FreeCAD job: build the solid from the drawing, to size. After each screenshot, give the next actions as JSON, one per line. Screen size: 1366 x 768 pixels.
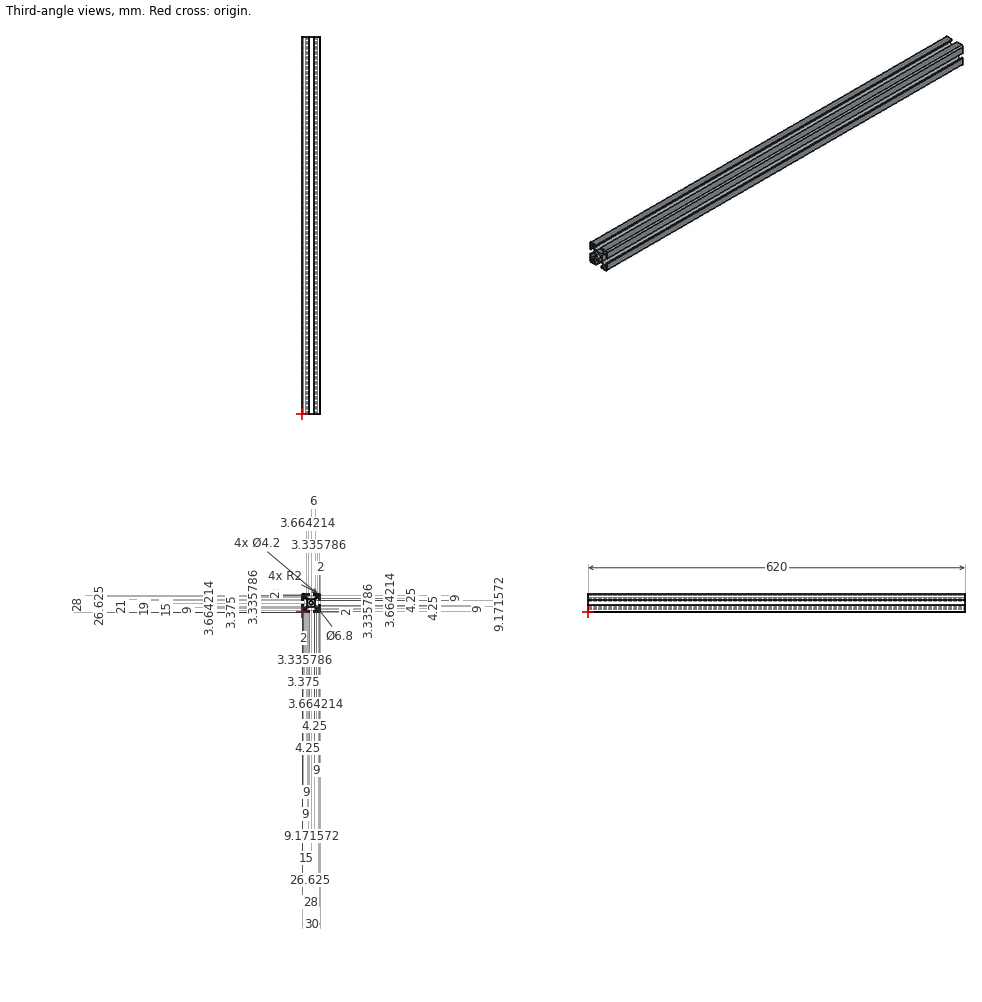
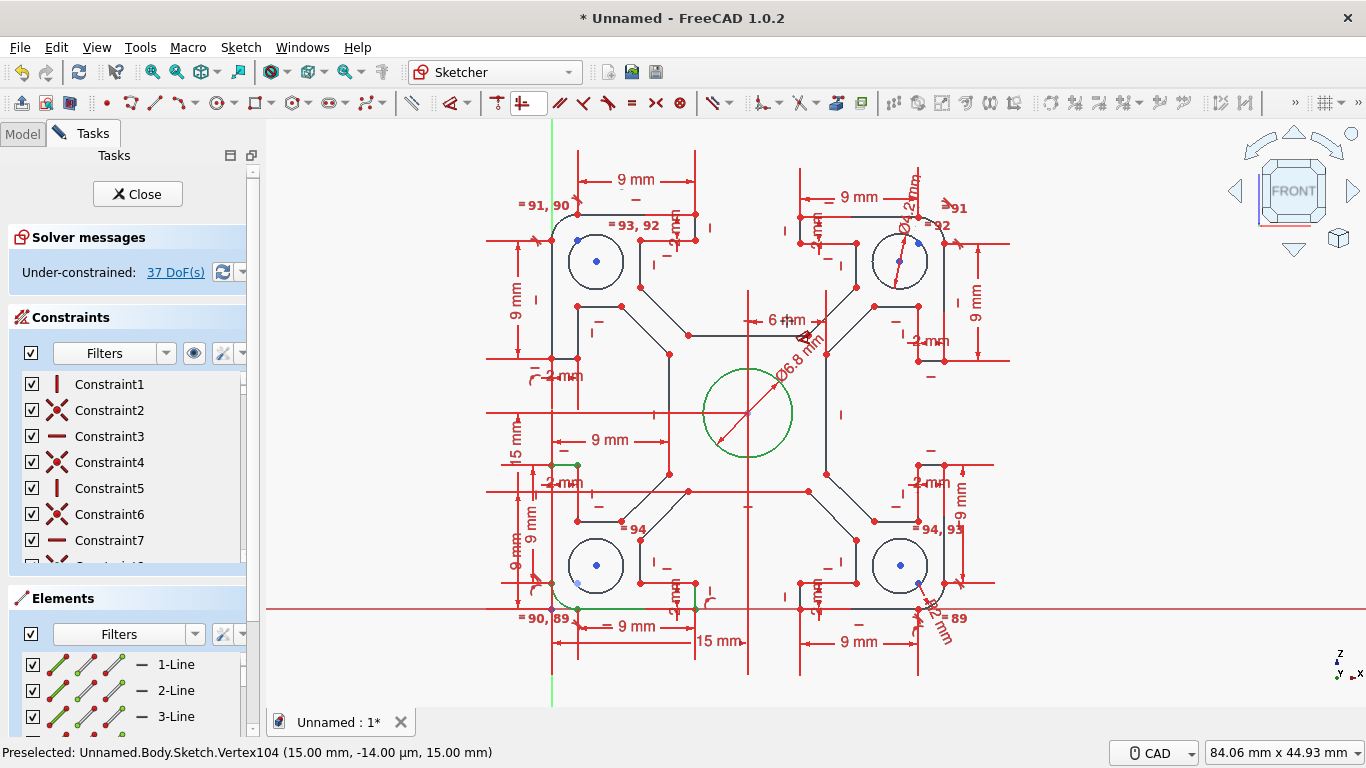
{"action": "left_click", "coordinate": [944, 244]}
{"action": "left_click", "coordinate": [748, 210]}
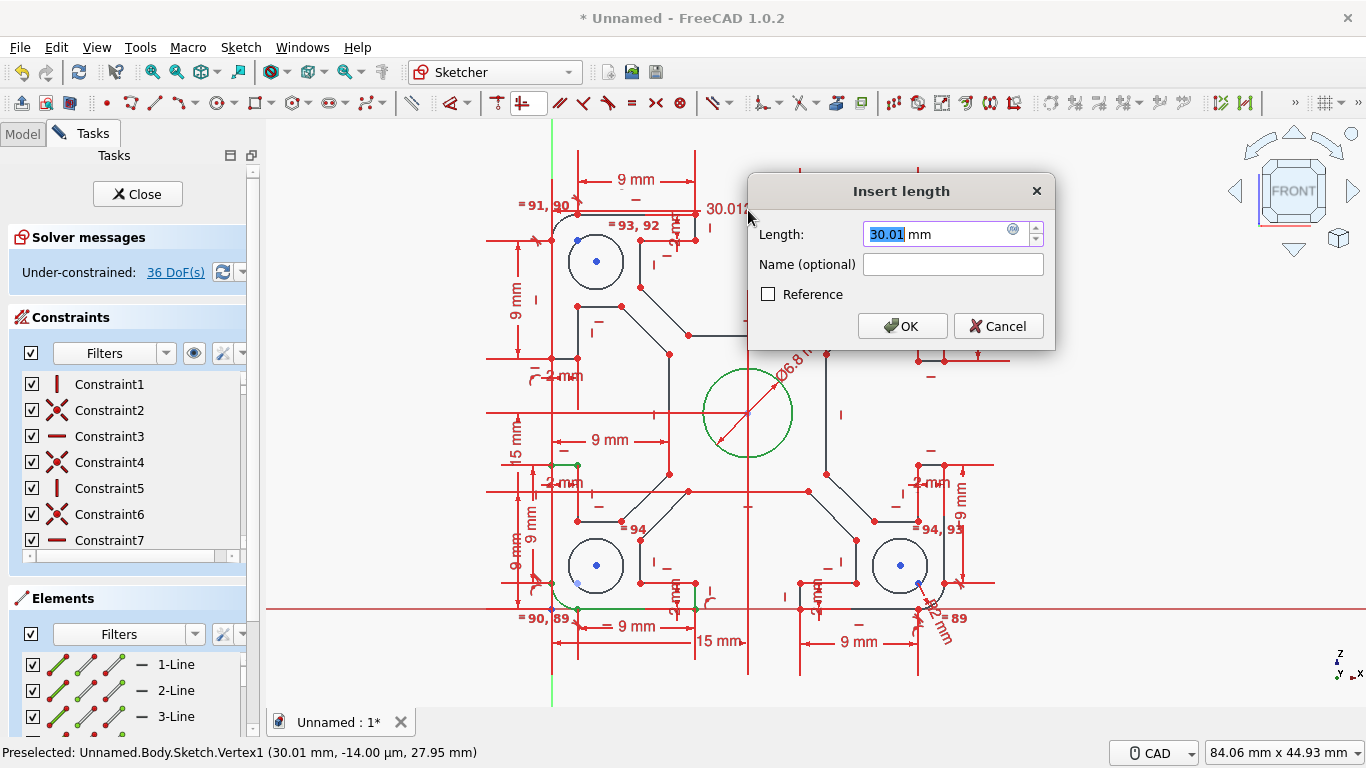
{"action": "type", "text": "30"}
{"action": "key", "text": "Return"}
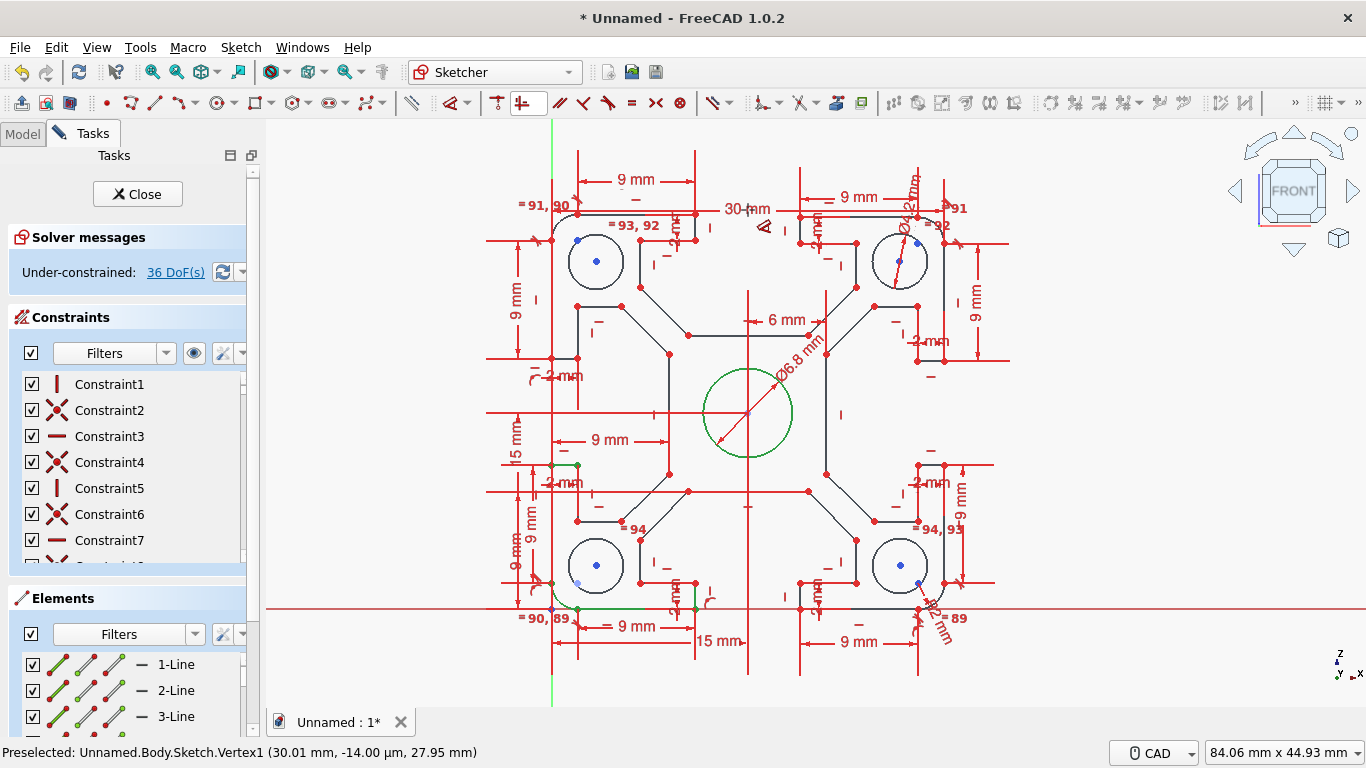
{"action": "left_click", "coordinate": [944, 244]}
{"action": "left_click", "coordinate": [518, 342]}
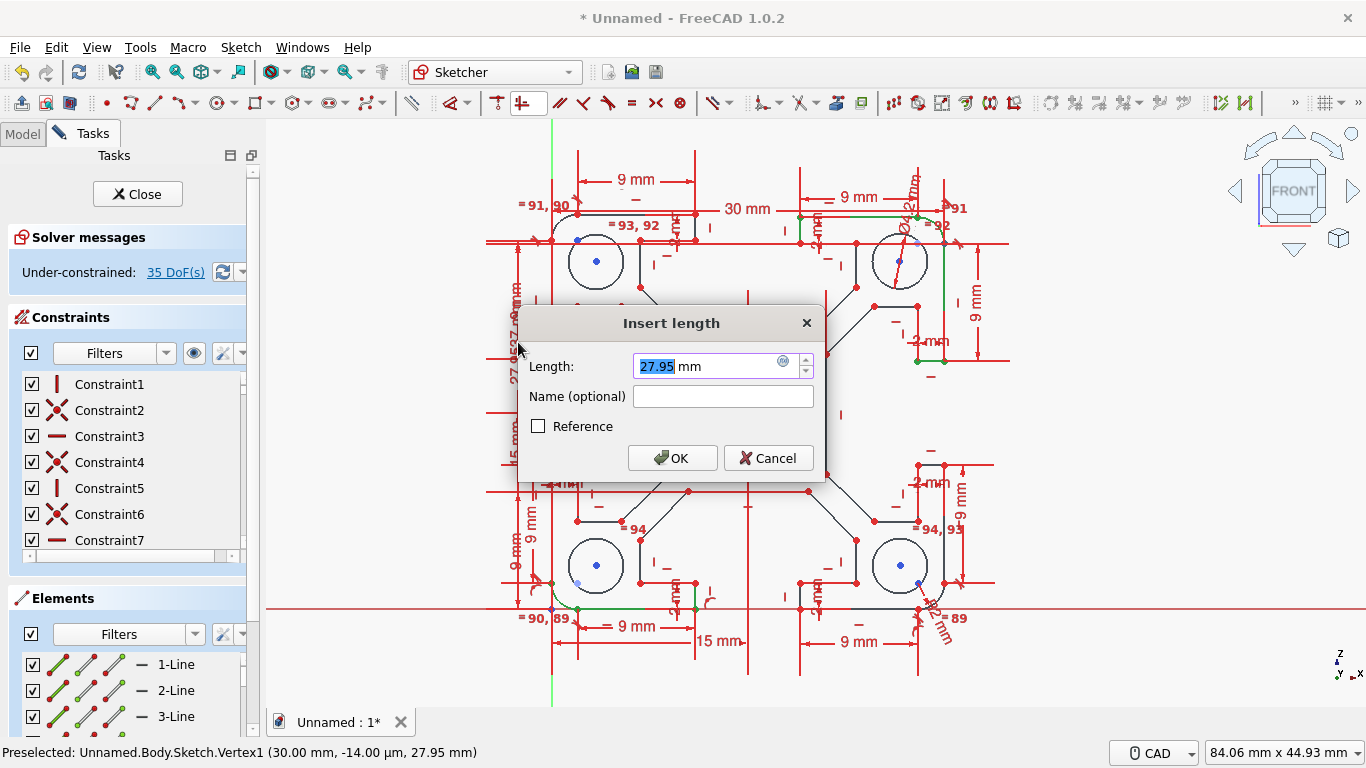
{"action": "type", "text": "28"}
{"action": "key", "text": "Return"}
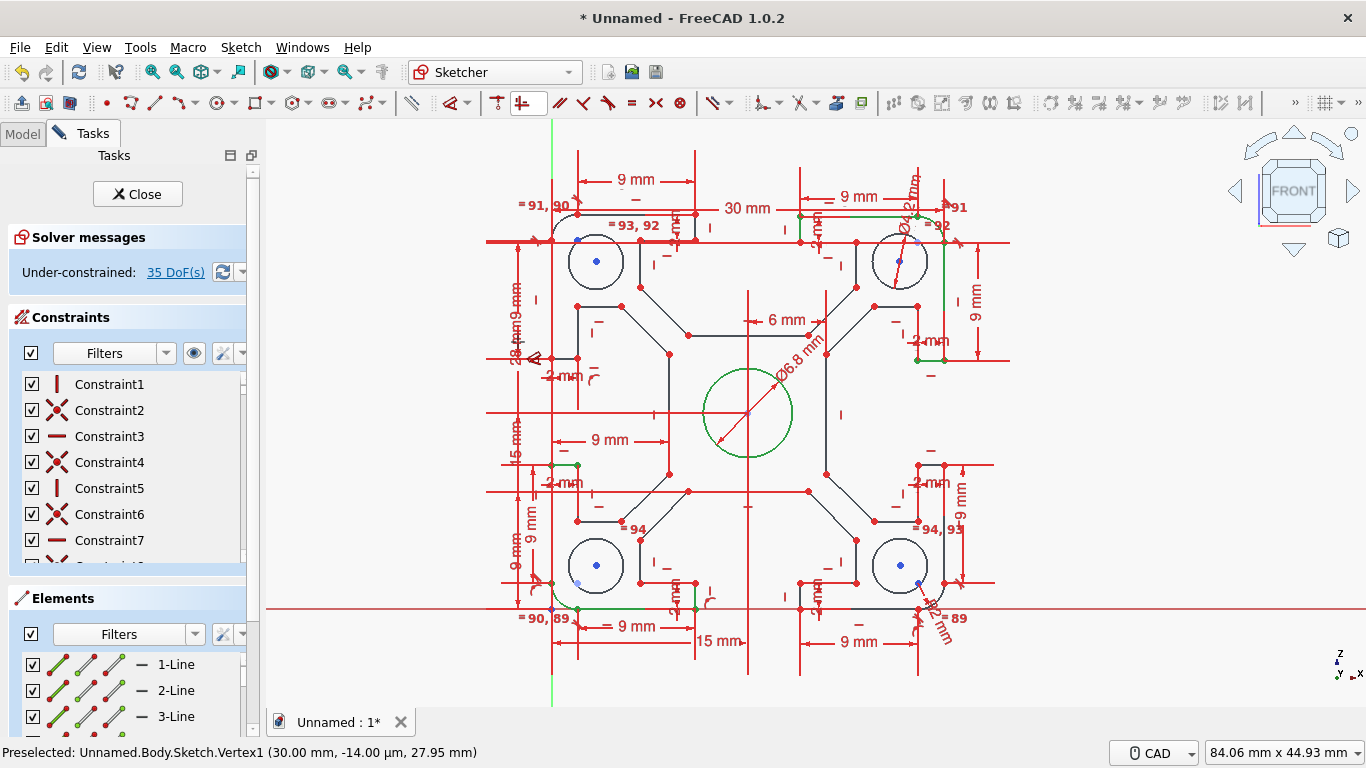
{"action": "left_click", "coordinate": [918, 522]}
{"action": "left_click", "coordinate": [735, 667]}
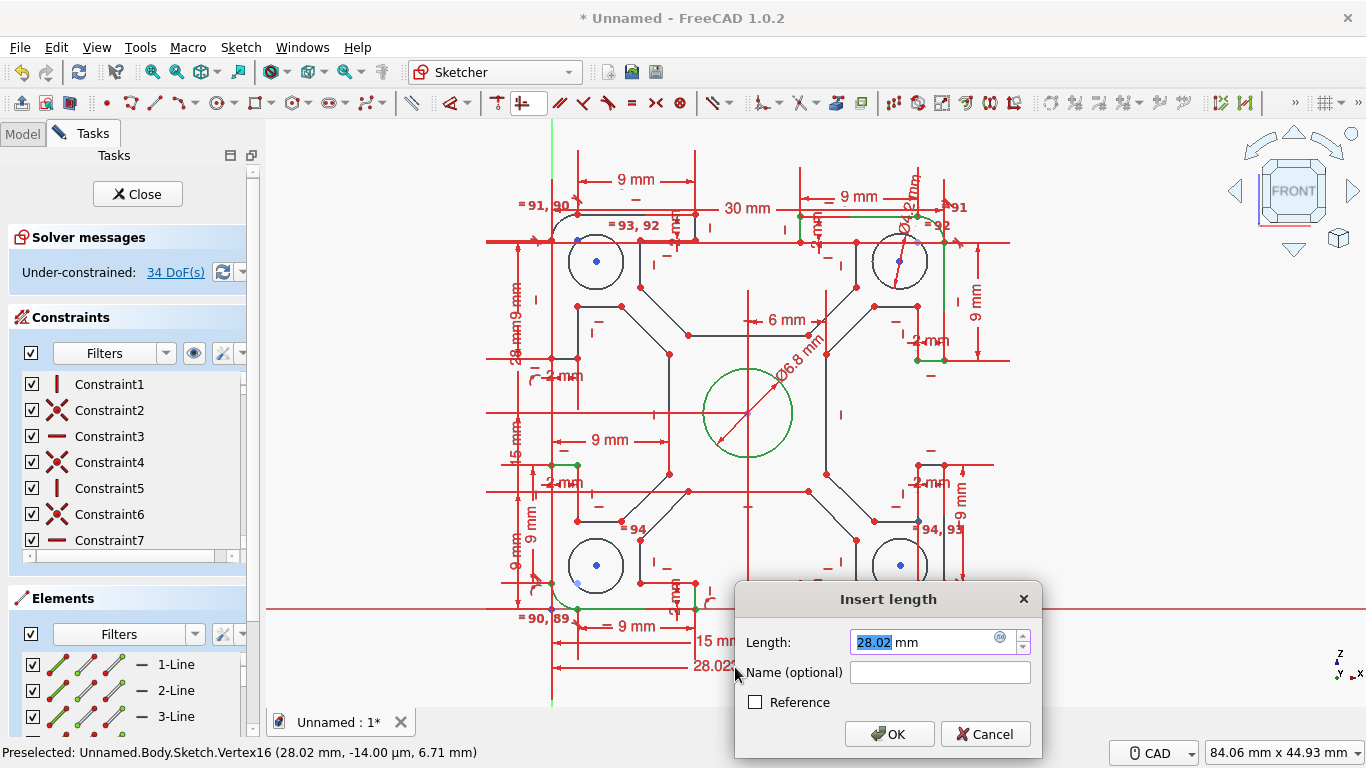
{"action": "type", "text": "28"}
{"action": "key", "text": "Return"}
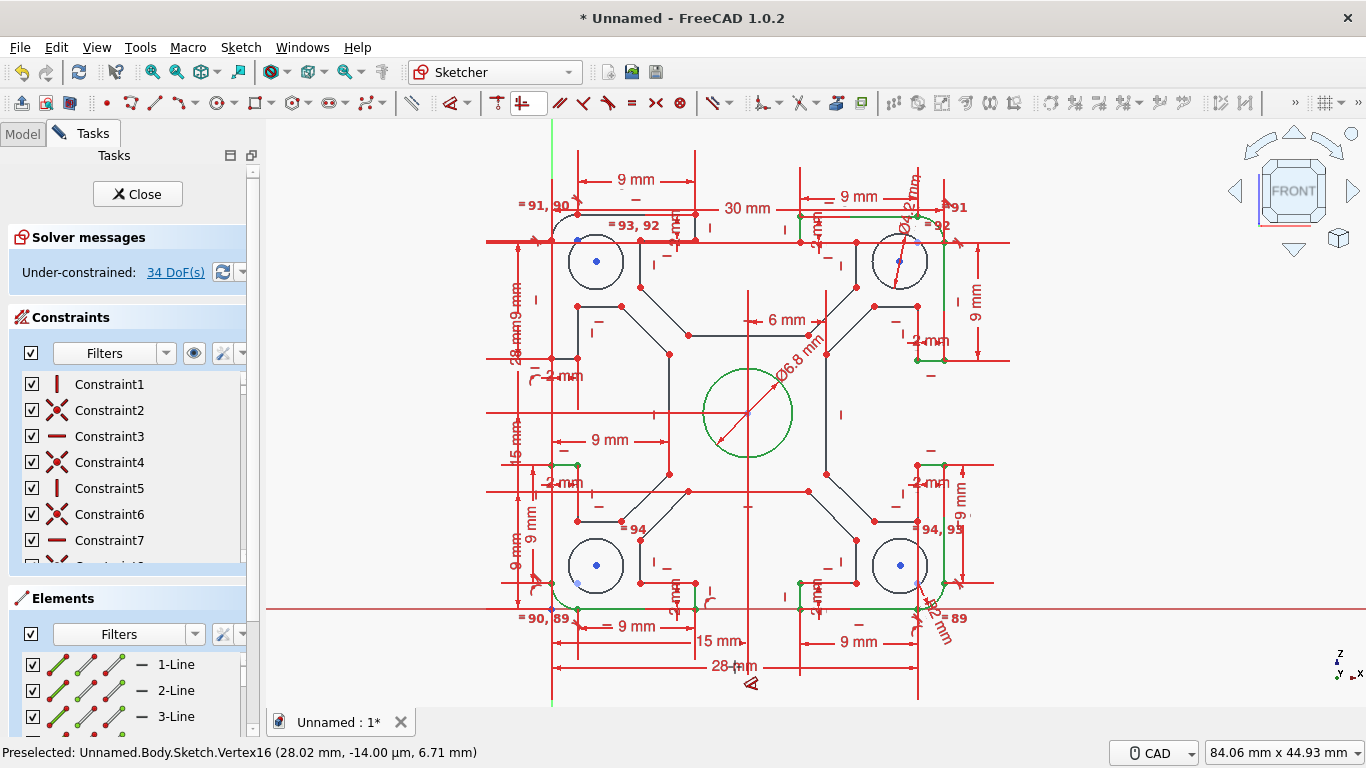
{"action": "left_click", "coordinate": [578, 359]}
{"action": "left_click", "coordinate": [518, 572]}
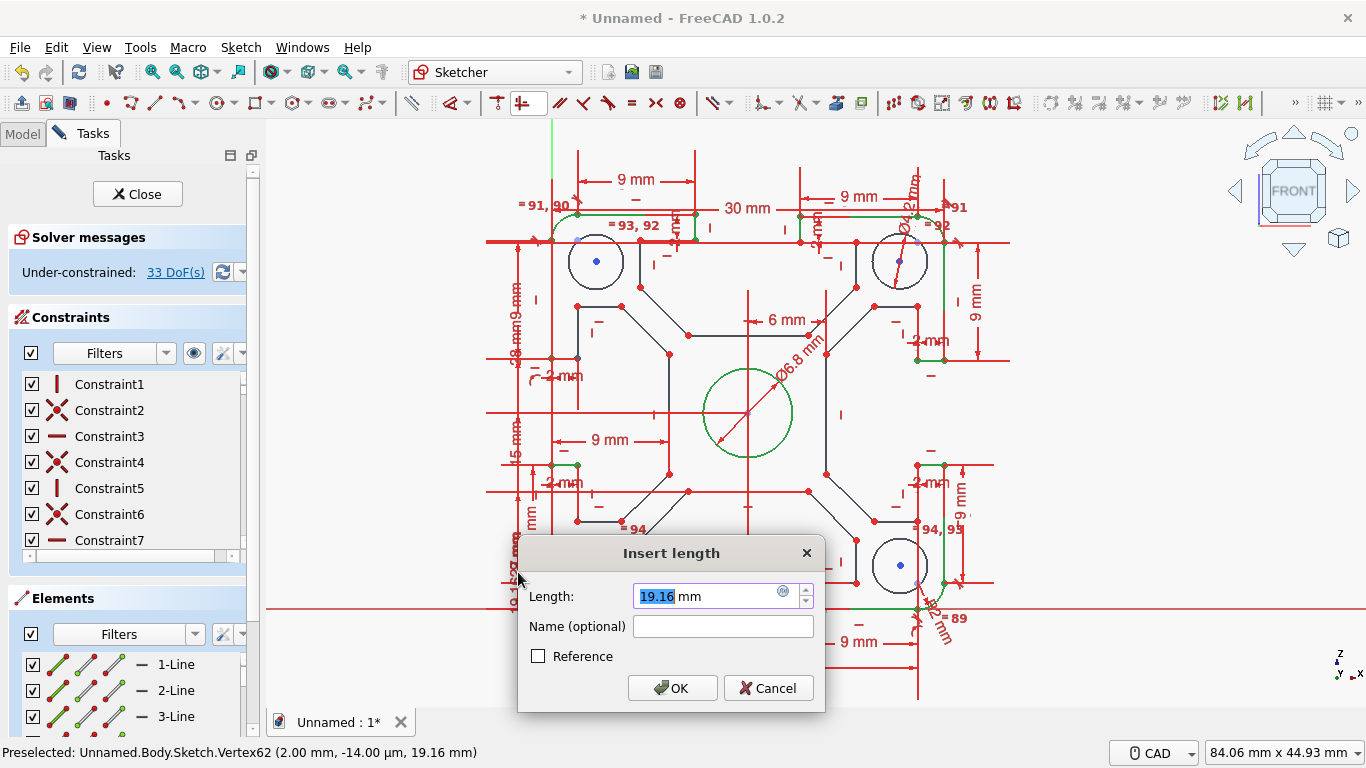
{"action": "type", "text": "19"}
{"action": "key", "text": "Return"}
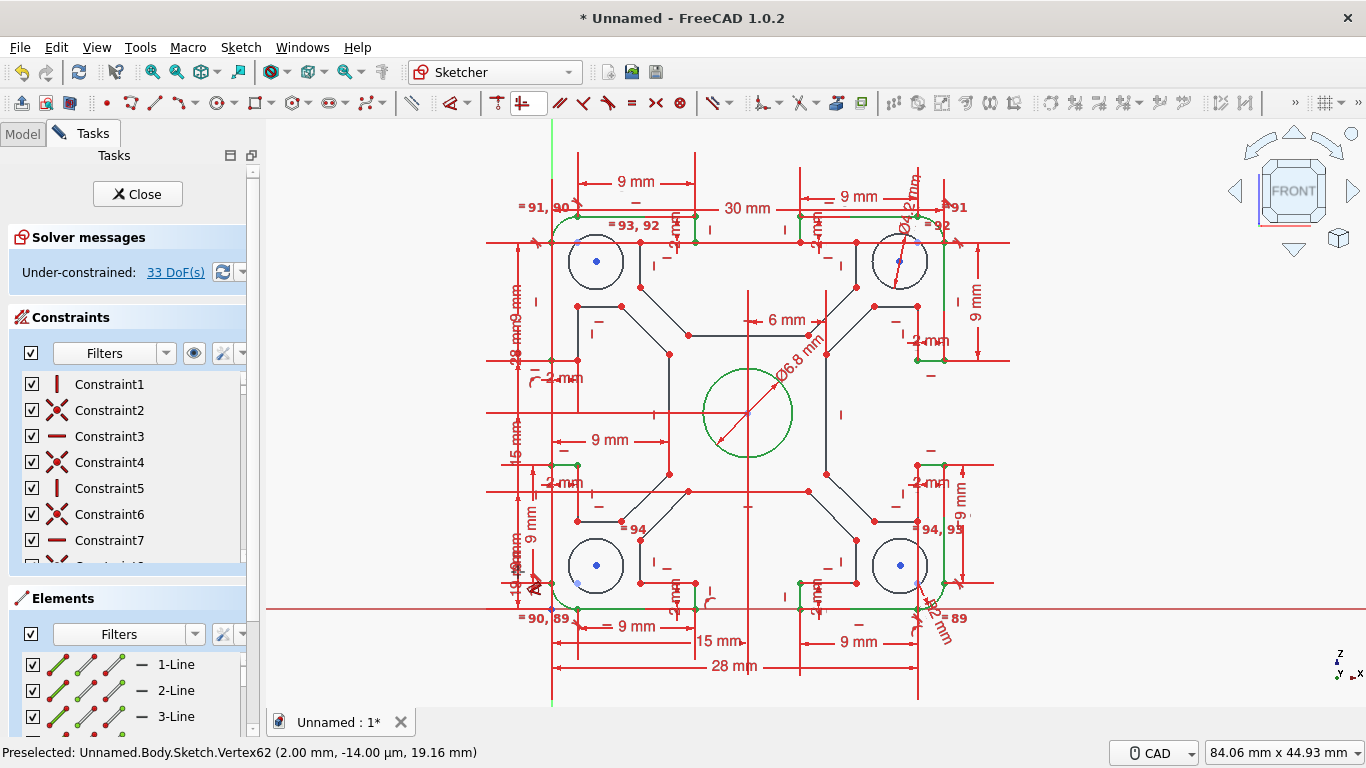
{"action": "left_click", "coordinate": [688, 336]}
{"action": "left_click", "coordinate": [518, 409]}